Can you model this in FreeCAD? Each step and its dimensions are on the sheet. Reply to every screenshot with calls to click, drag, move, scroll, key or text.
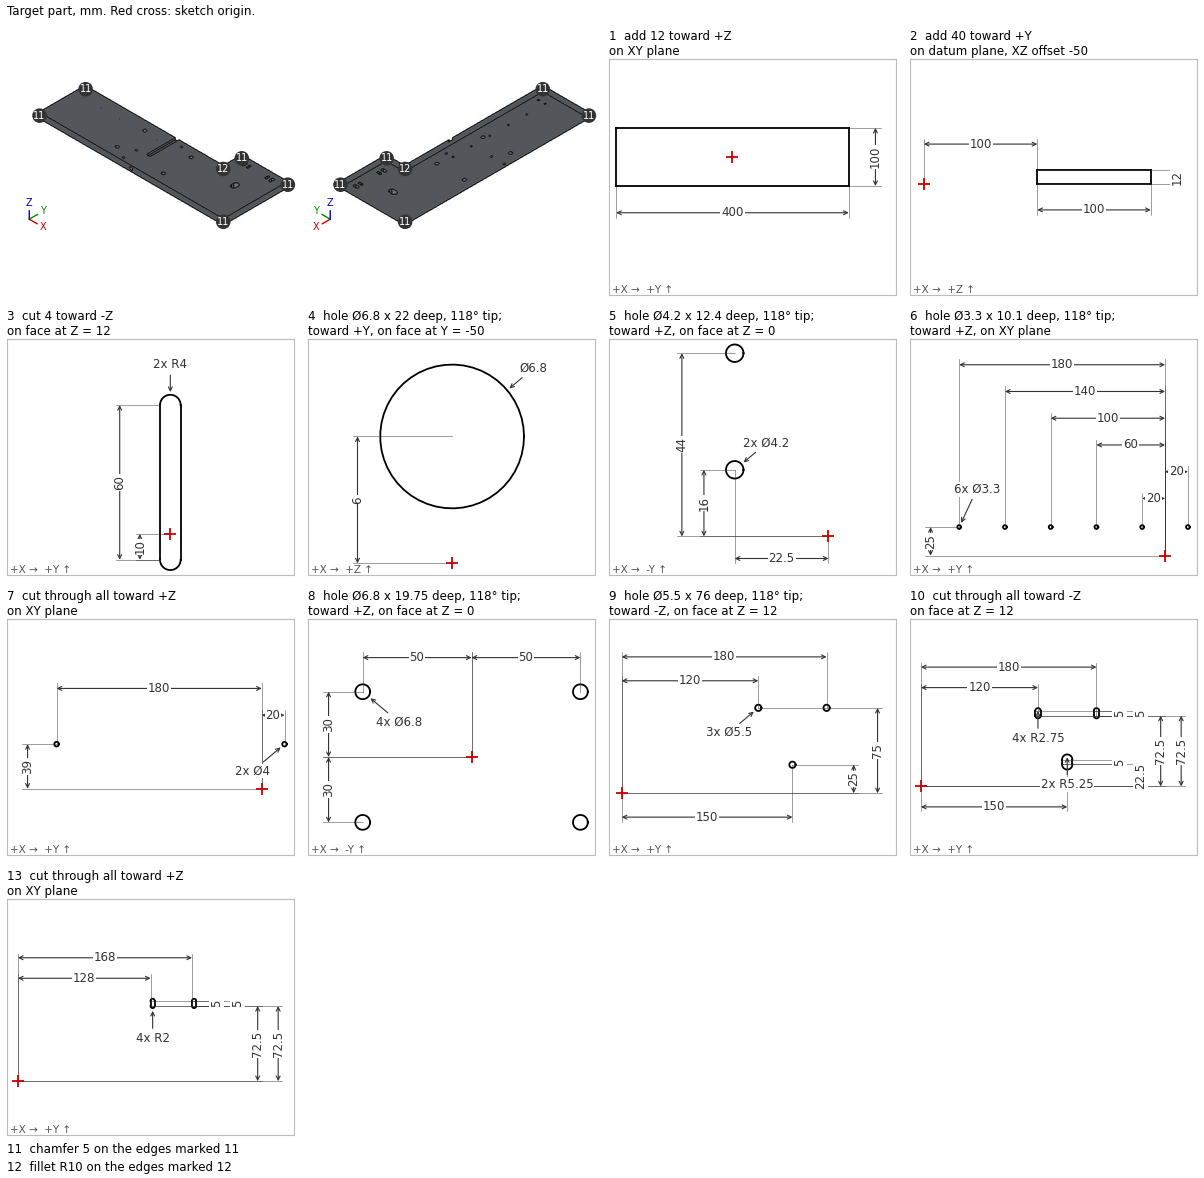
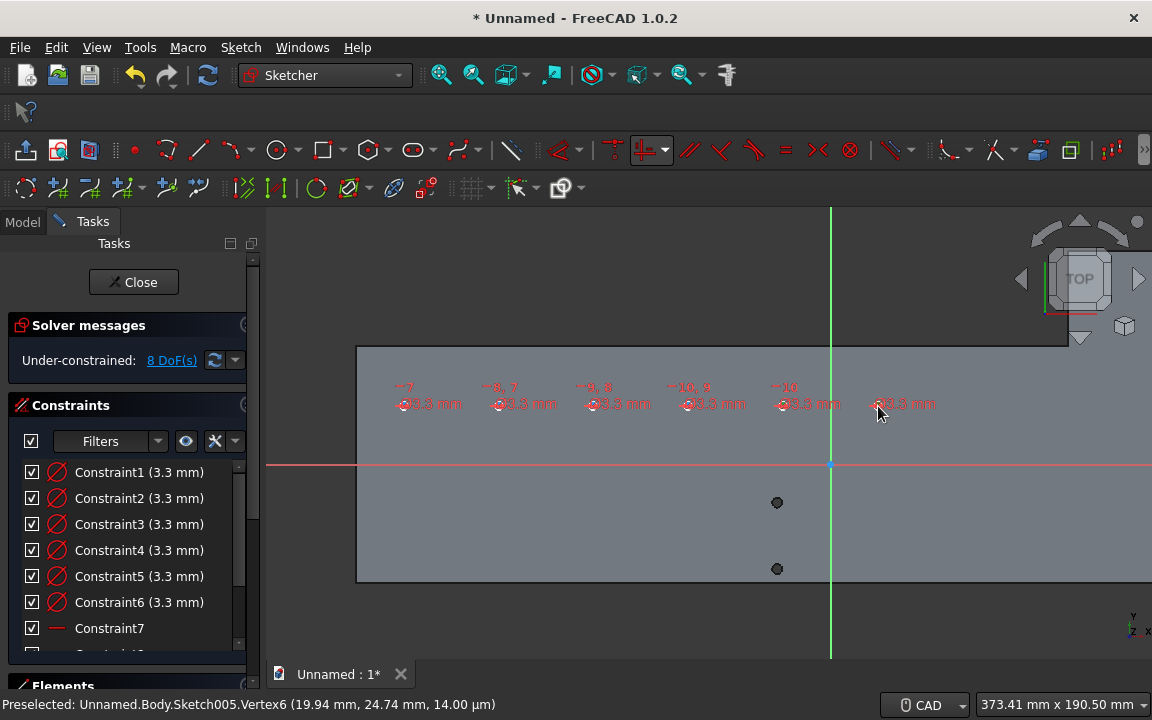
click(668, 150)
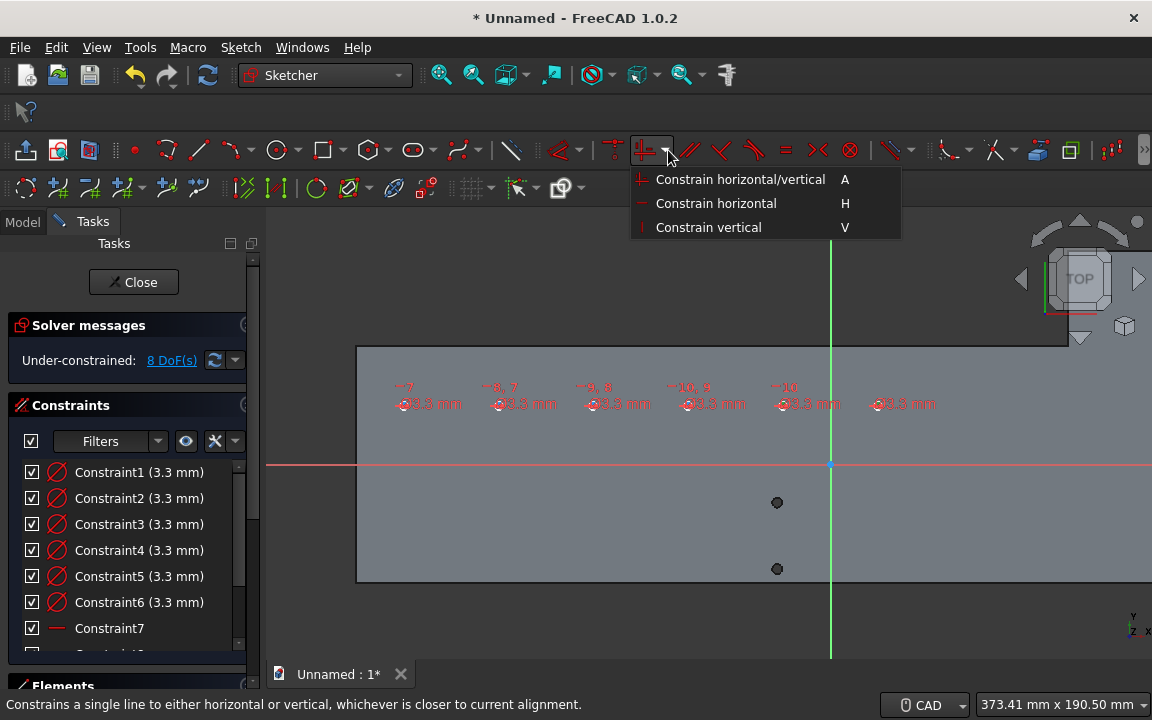
click(766, 203)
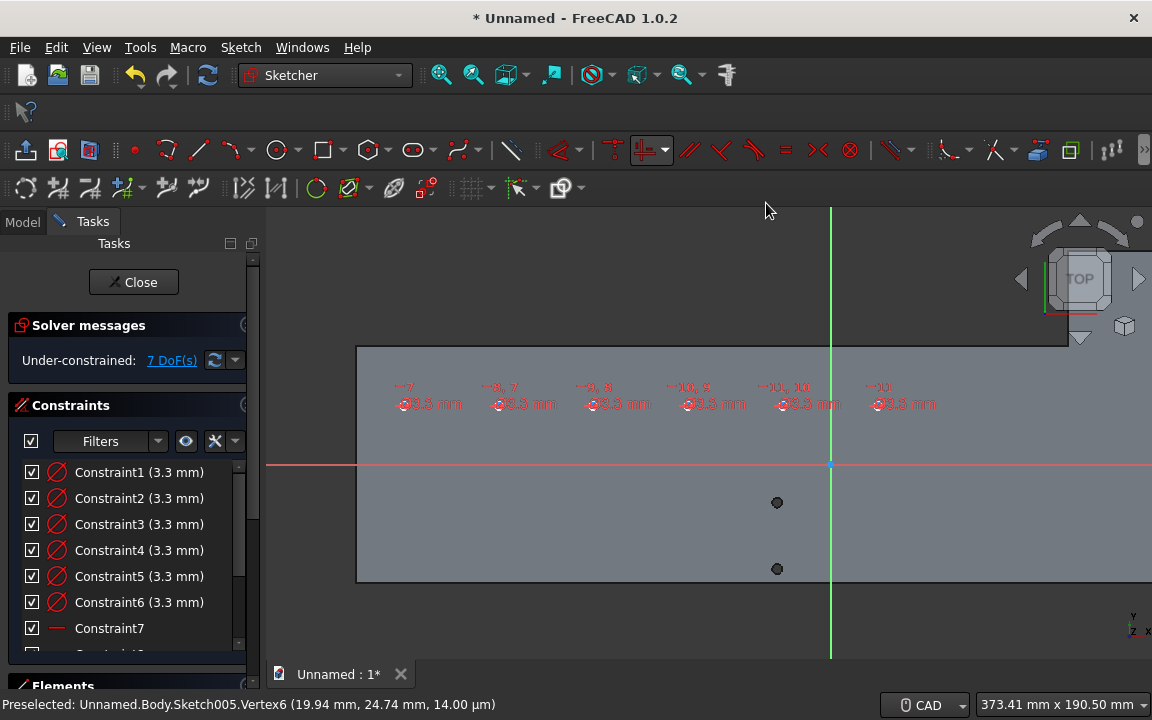
click(558, 150)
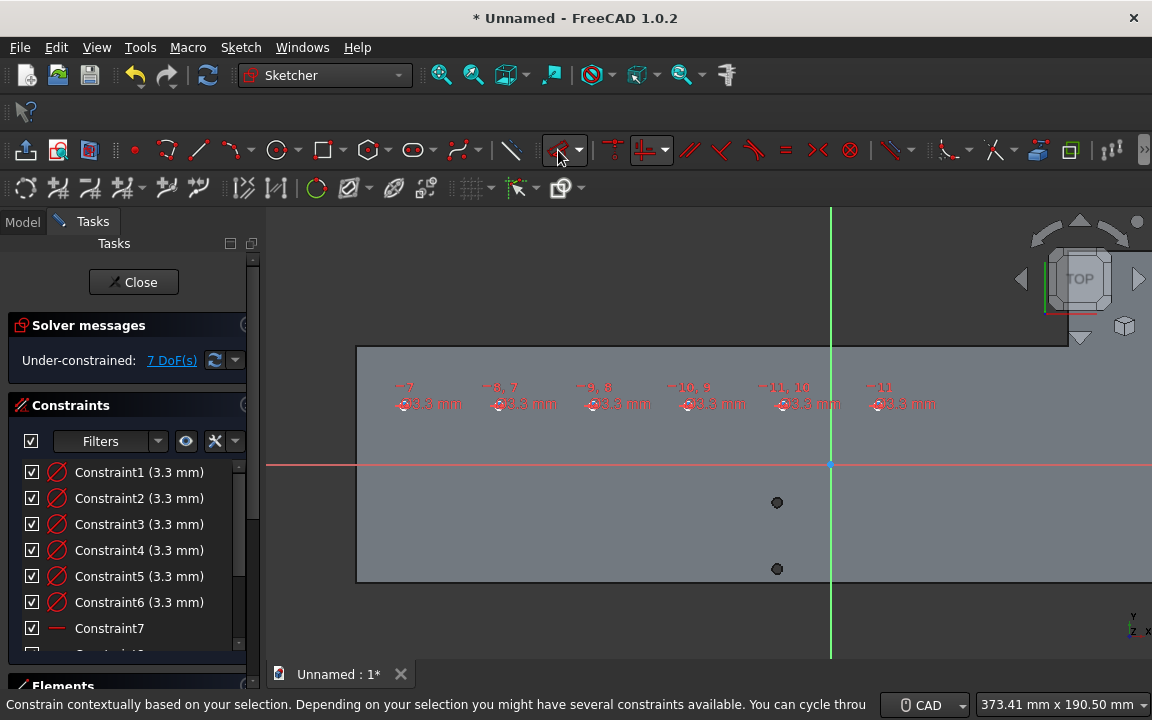
click(404, 406)
click(370, 435)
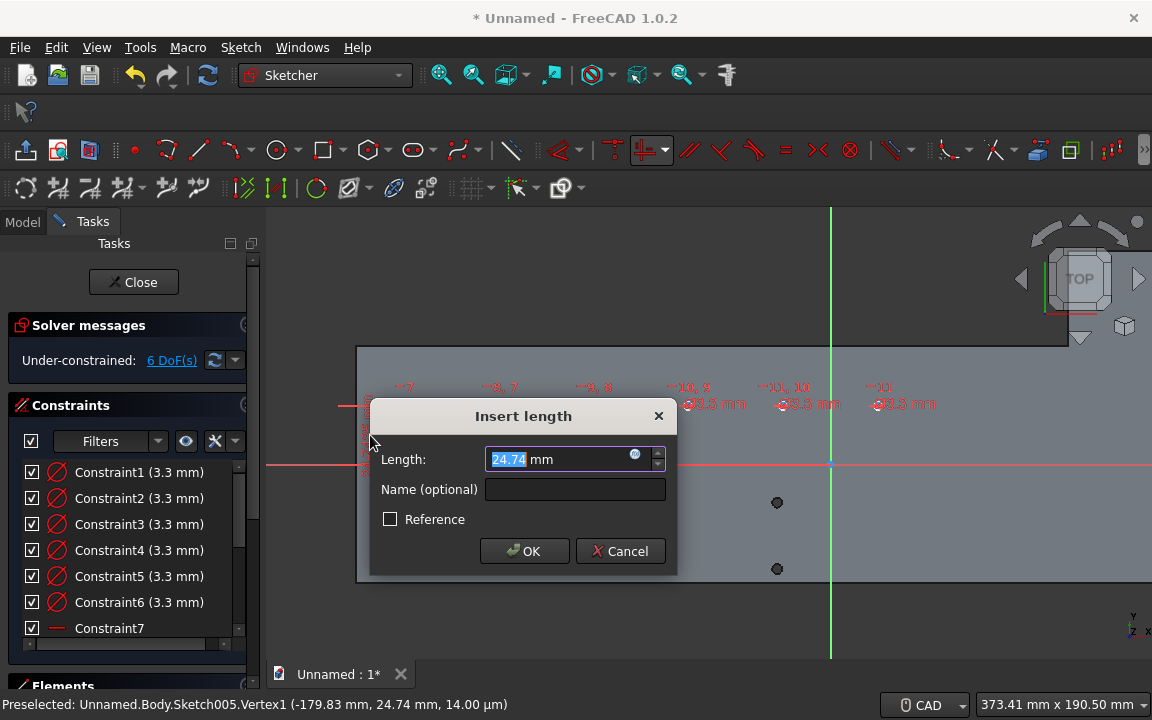
text(25)
key(Return)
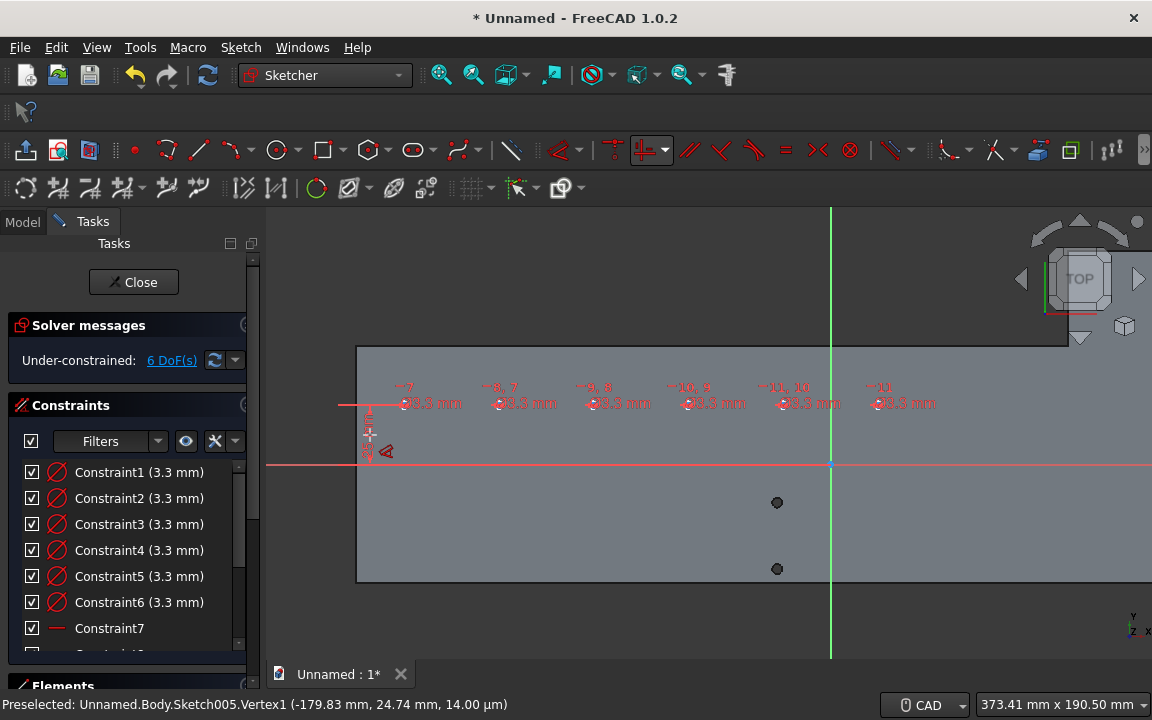
click(688, 405)
click(759, 499)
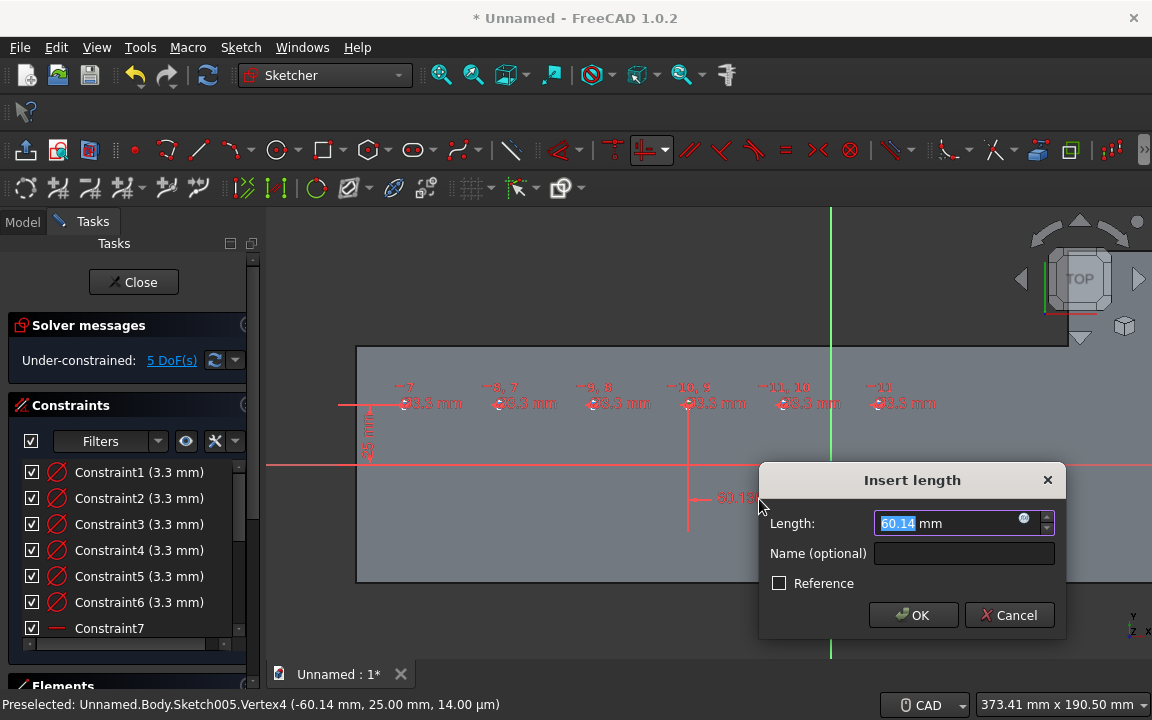
text(60)
key(Return)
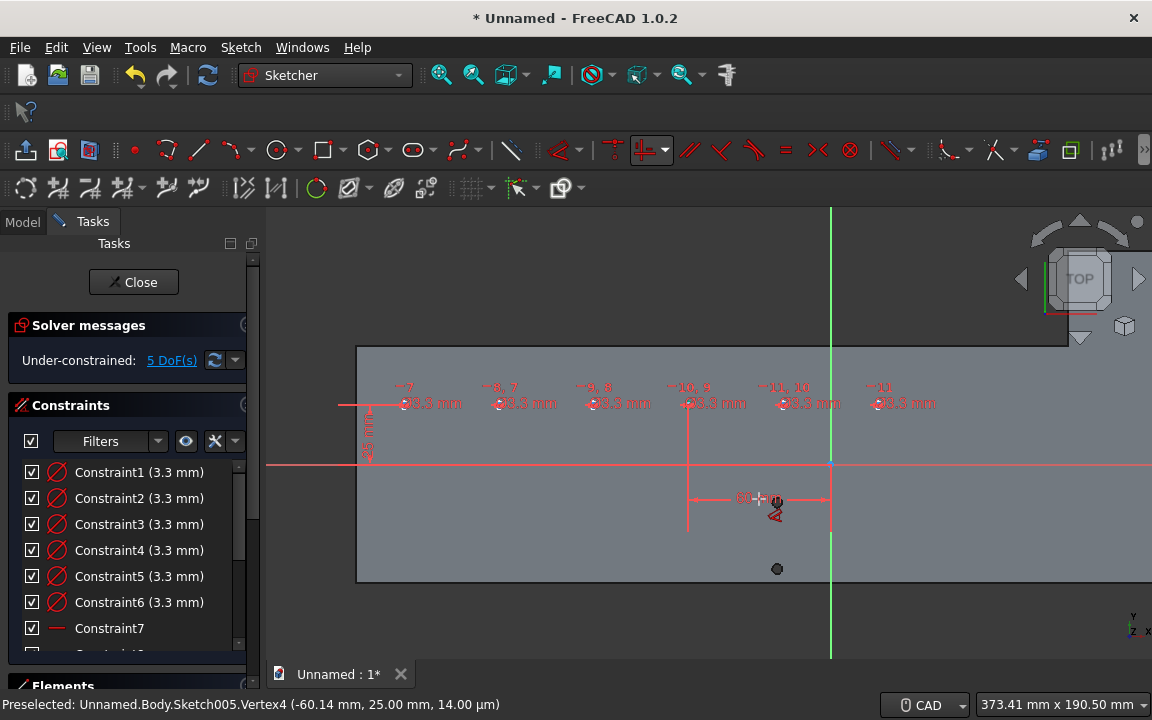
click(783, 405)
click(807, 371)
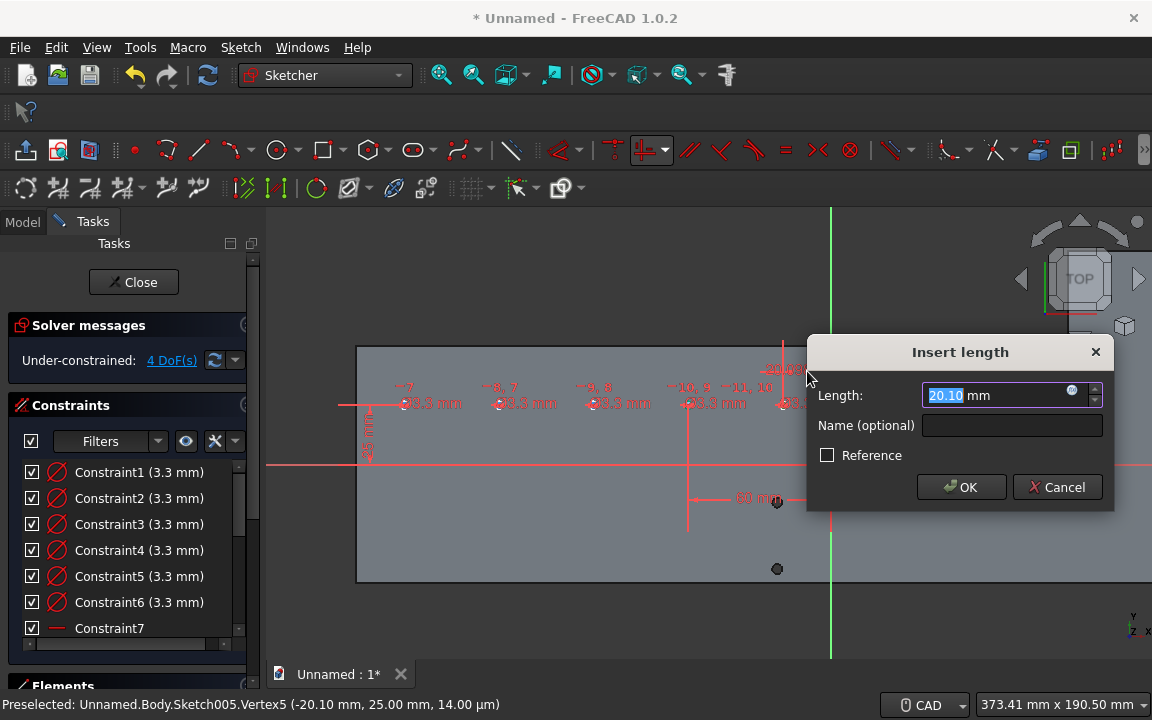
text(20)
key(Return)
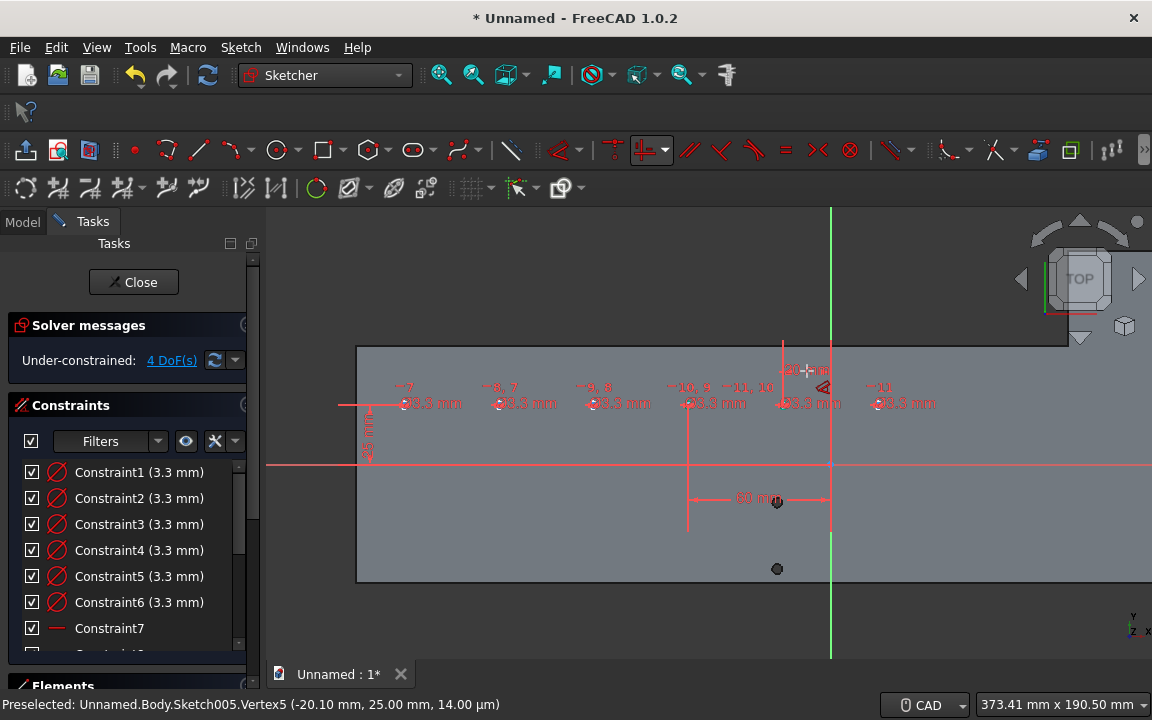
click(878, 405)
click(854, 499)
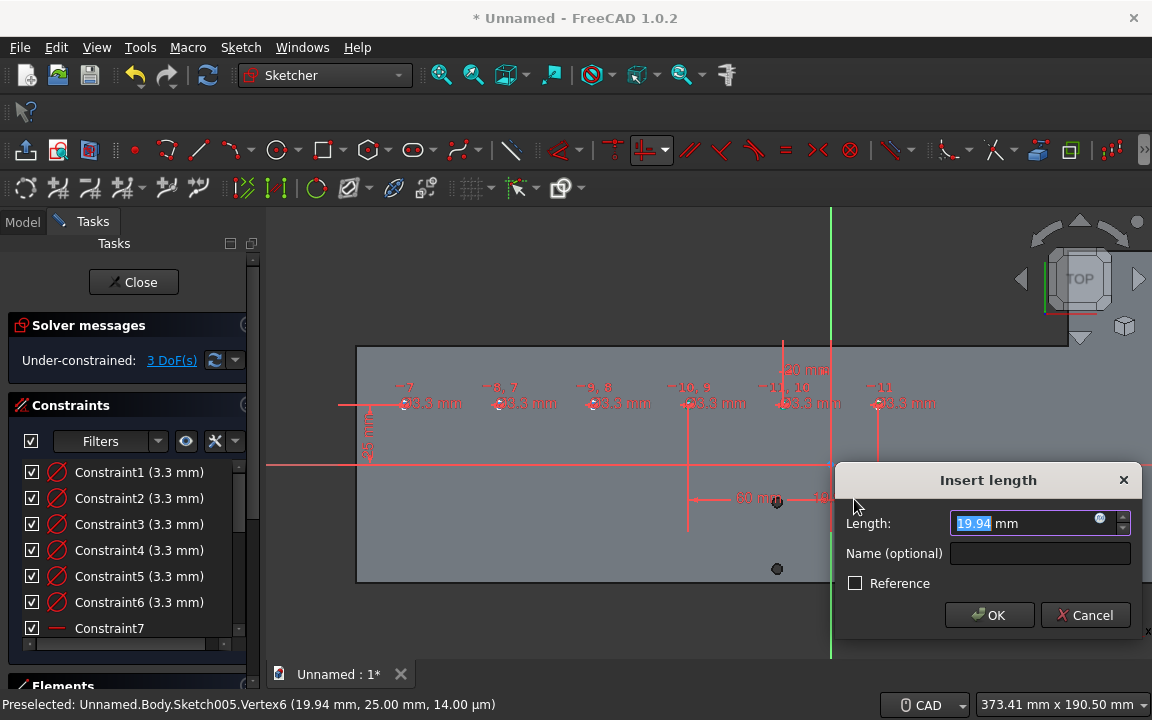
text(20)
key(Return)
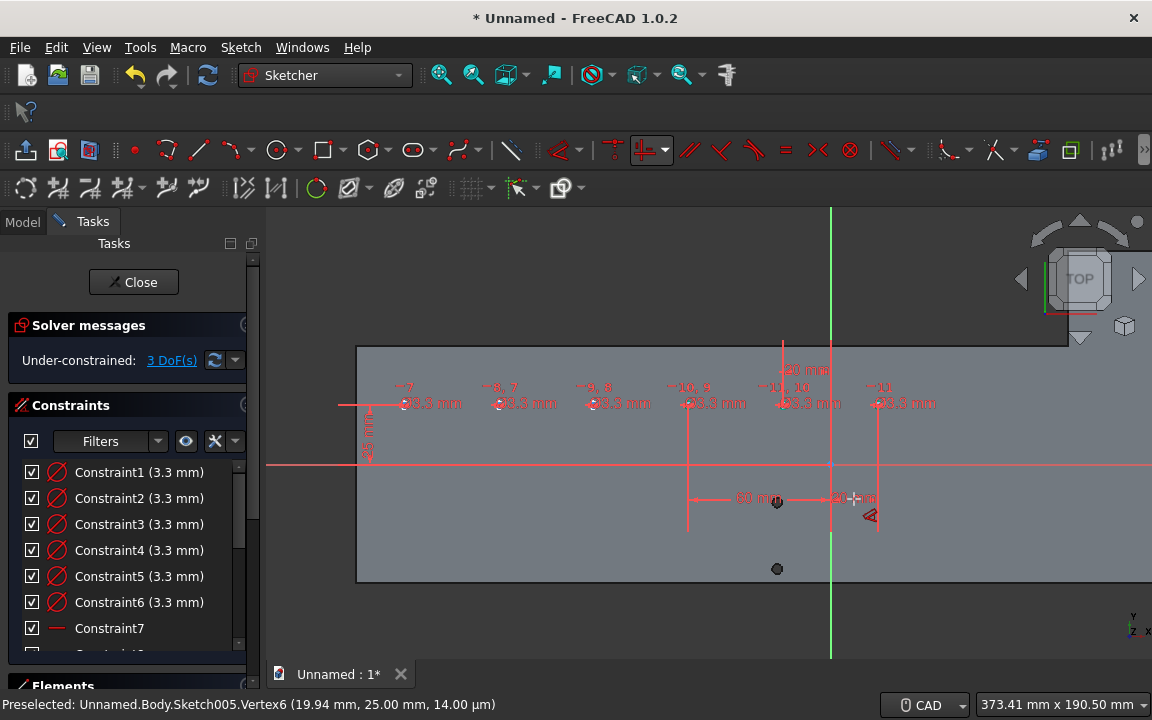
click(404, 405)
click(617, 499)